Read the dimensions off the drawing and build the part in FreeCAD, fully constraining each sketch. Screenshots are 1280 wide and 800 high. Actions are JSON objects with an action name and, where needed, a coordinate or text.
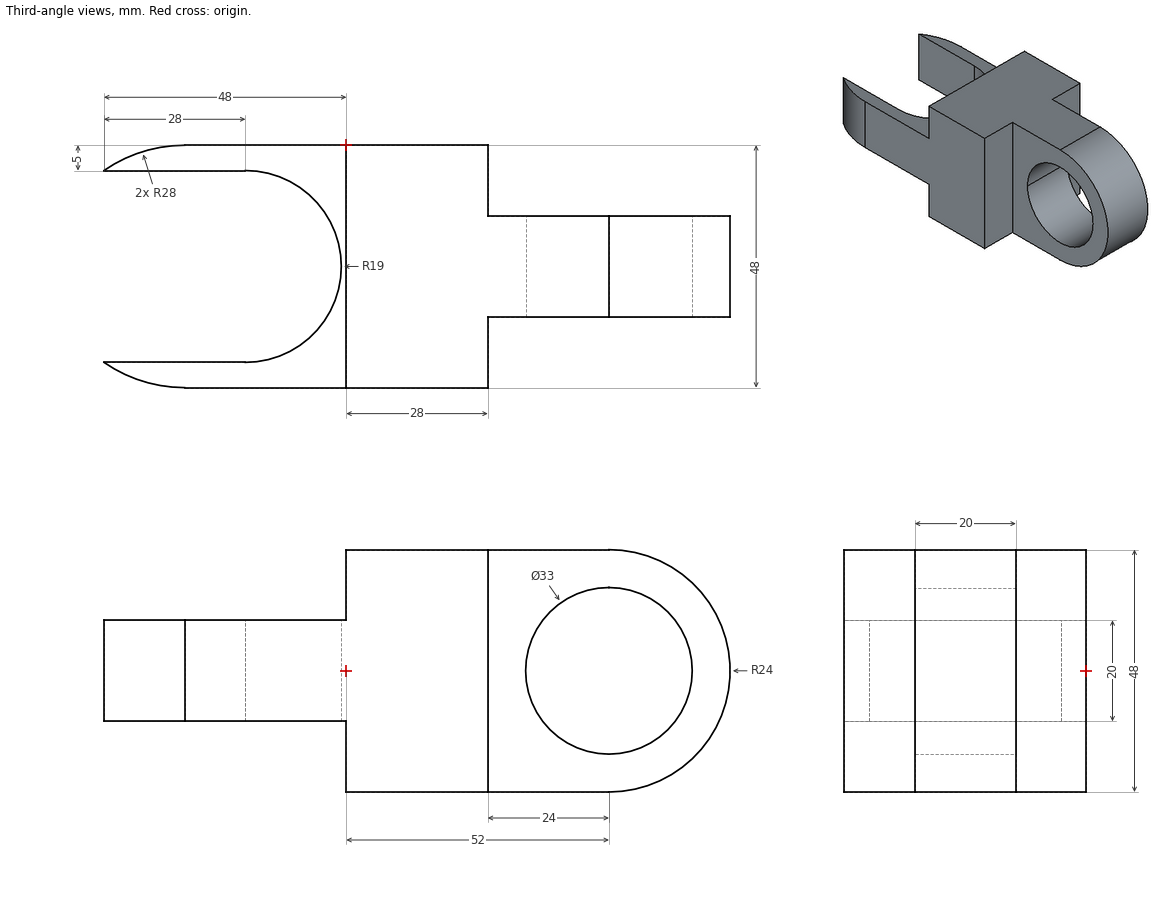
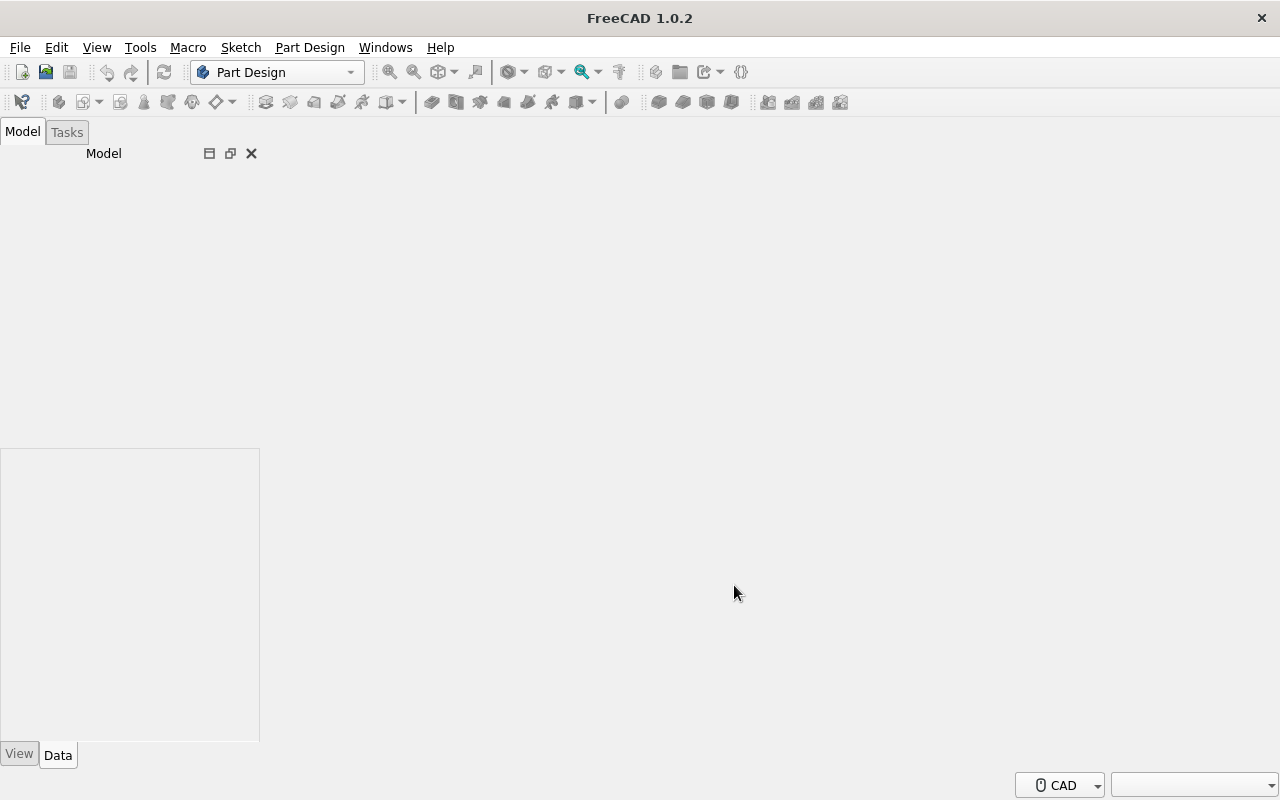
{"action": "left_click", "coordinate": [22, 72]}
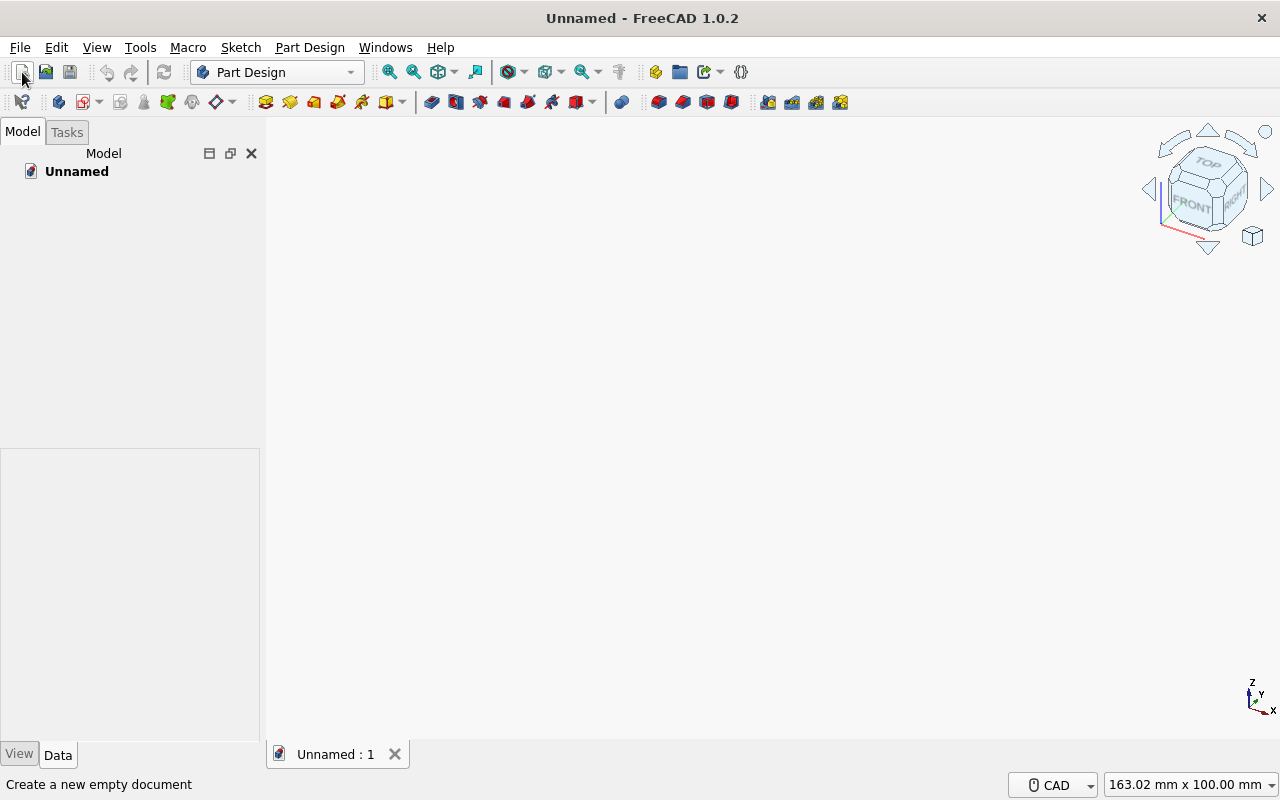
{"action": "left_click", "coordinate": [84, 102]}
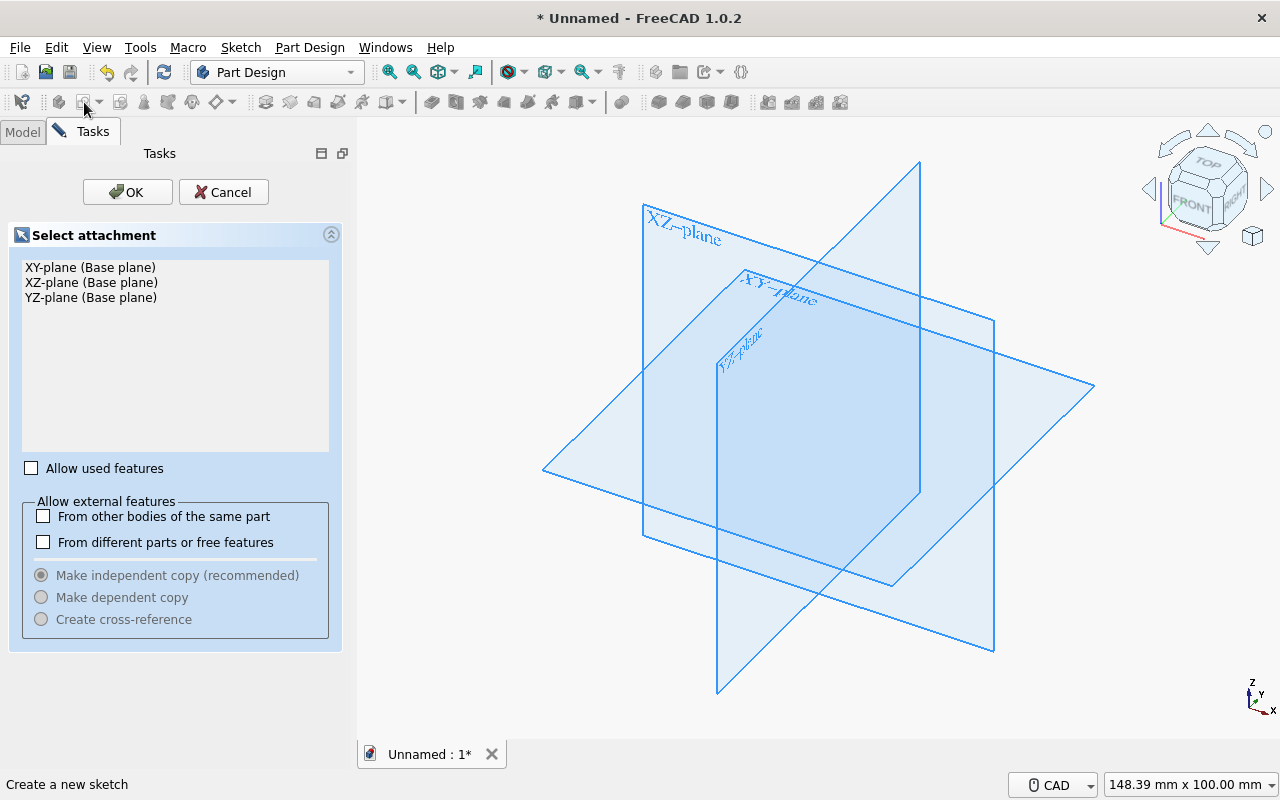
{"action": "left_click", "coordinate": [82, 268]}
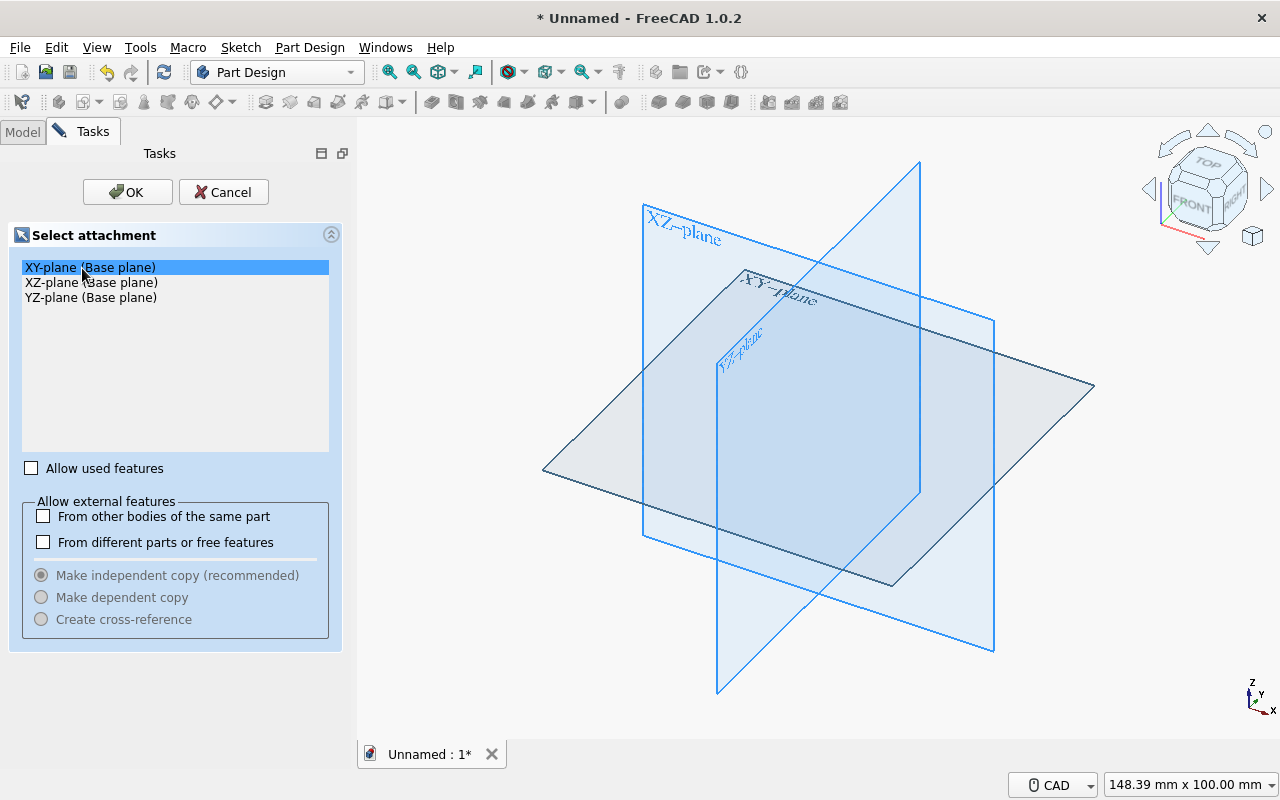
{"action": "left_click", "coordinate": [128, 192]}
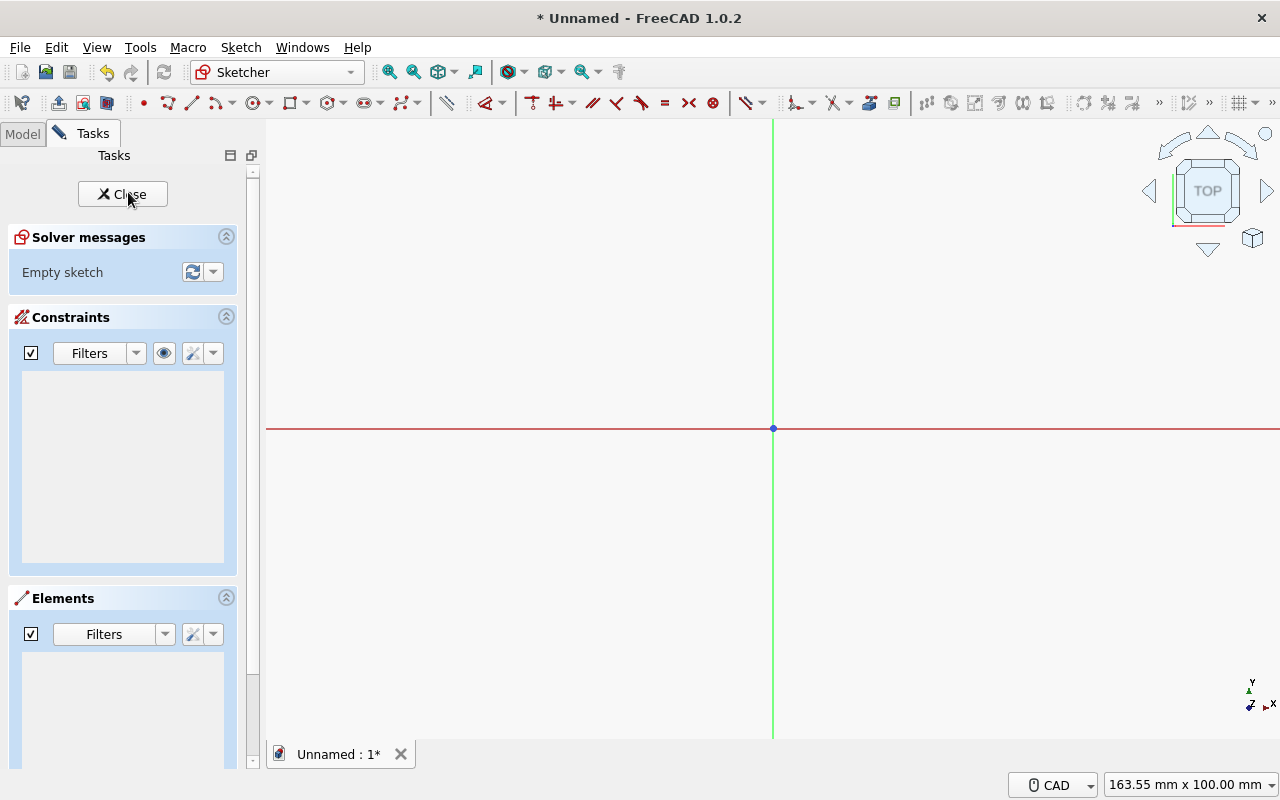
{"action": "scroll", "coordinate": [294, 147], "scroll_direction": "down", "scroll_amount": 1}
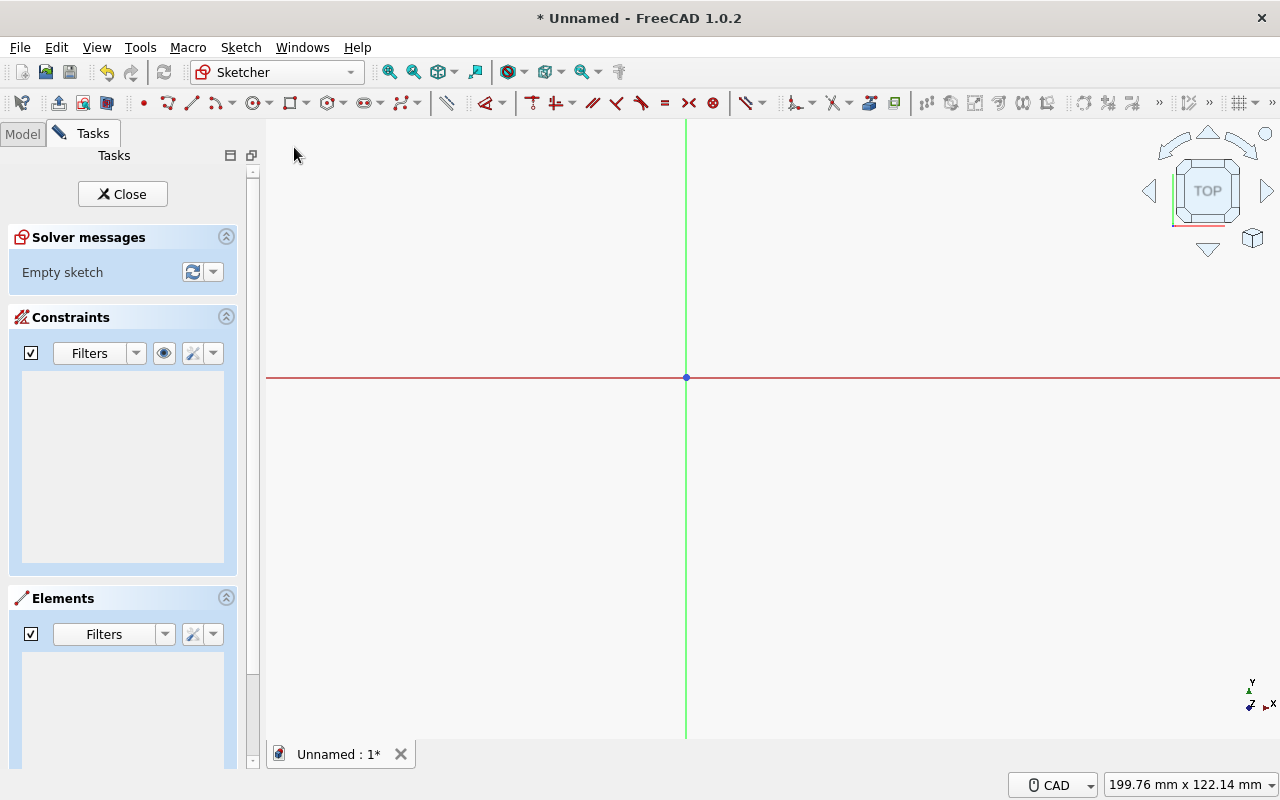
{"action": "scroll", "coordinate": [864, 644], "scroll_direction": "up", "scroll_amount": 2}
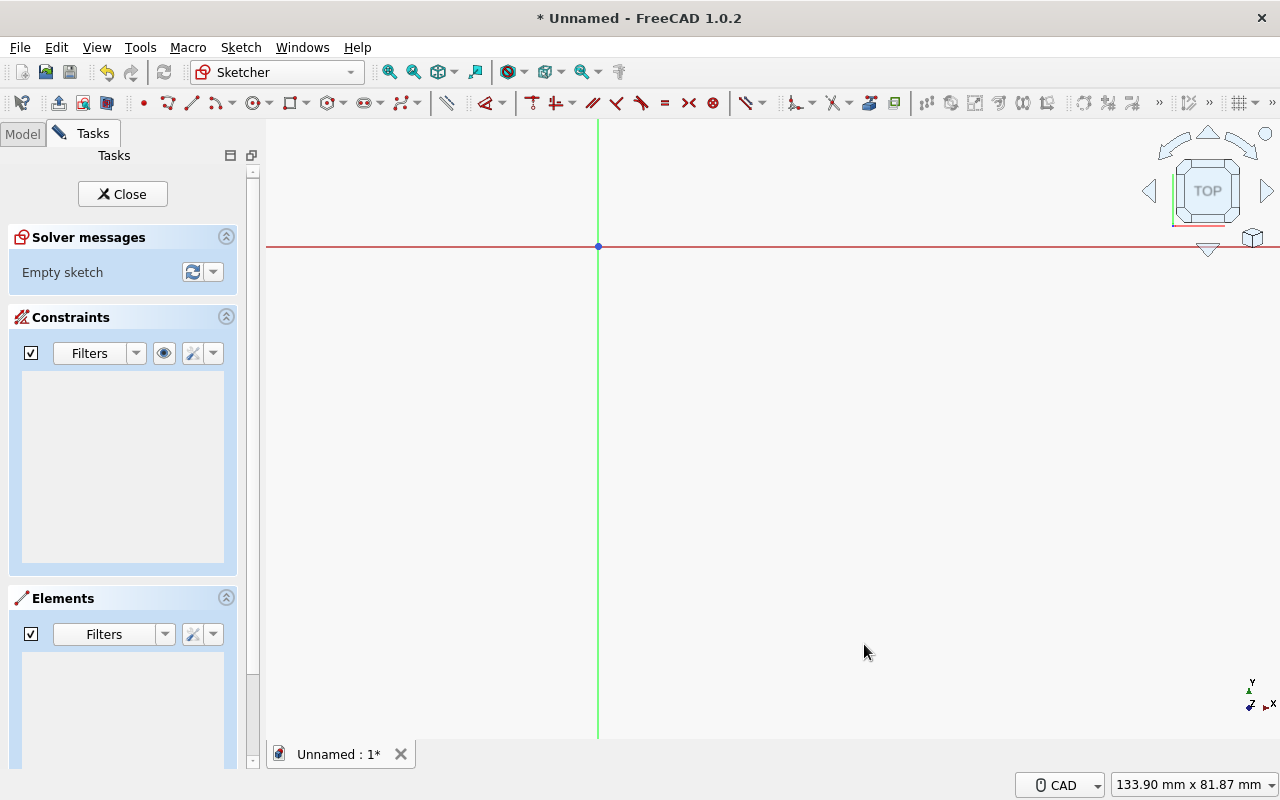
{"action": "left_click", "coordinate": [290, 104]}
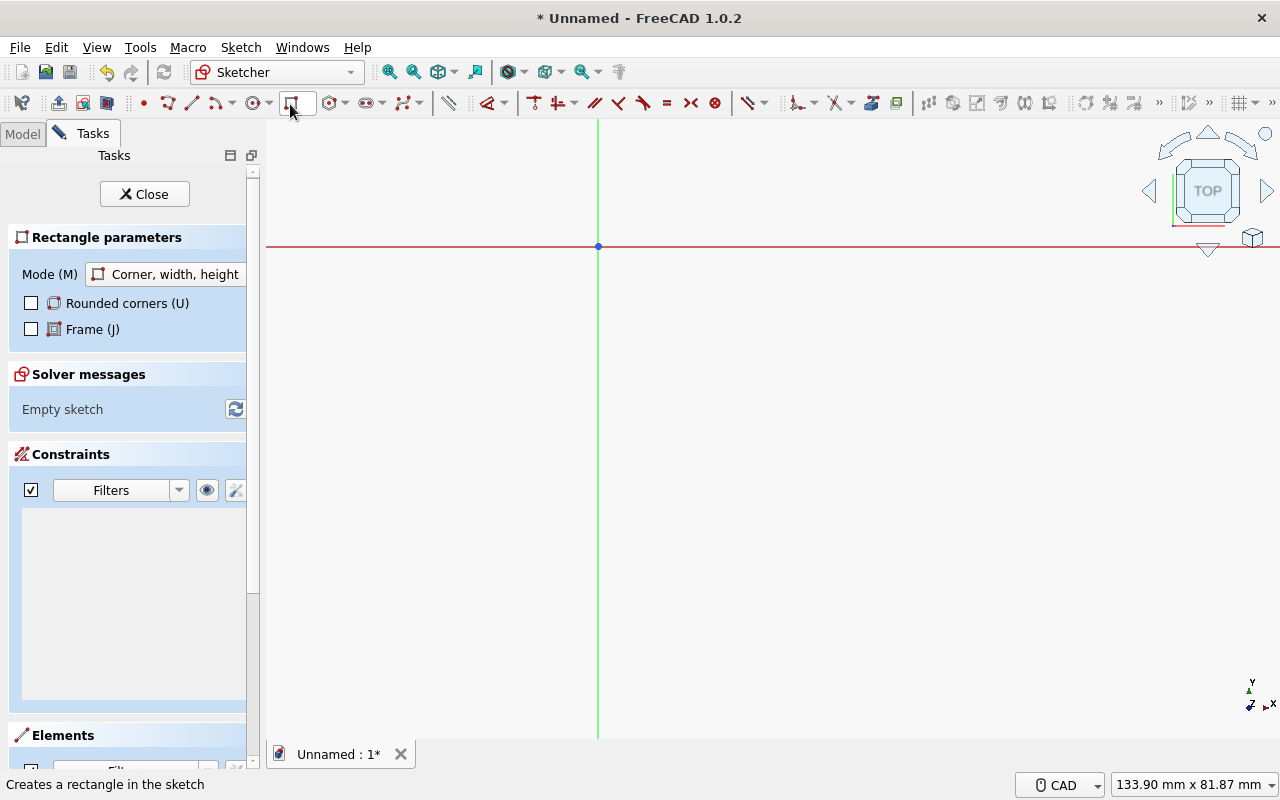
{"action": "left_click", "coordinate": [598, 247]}
{"action": "mouse_move", "coordinate": [810, 610]}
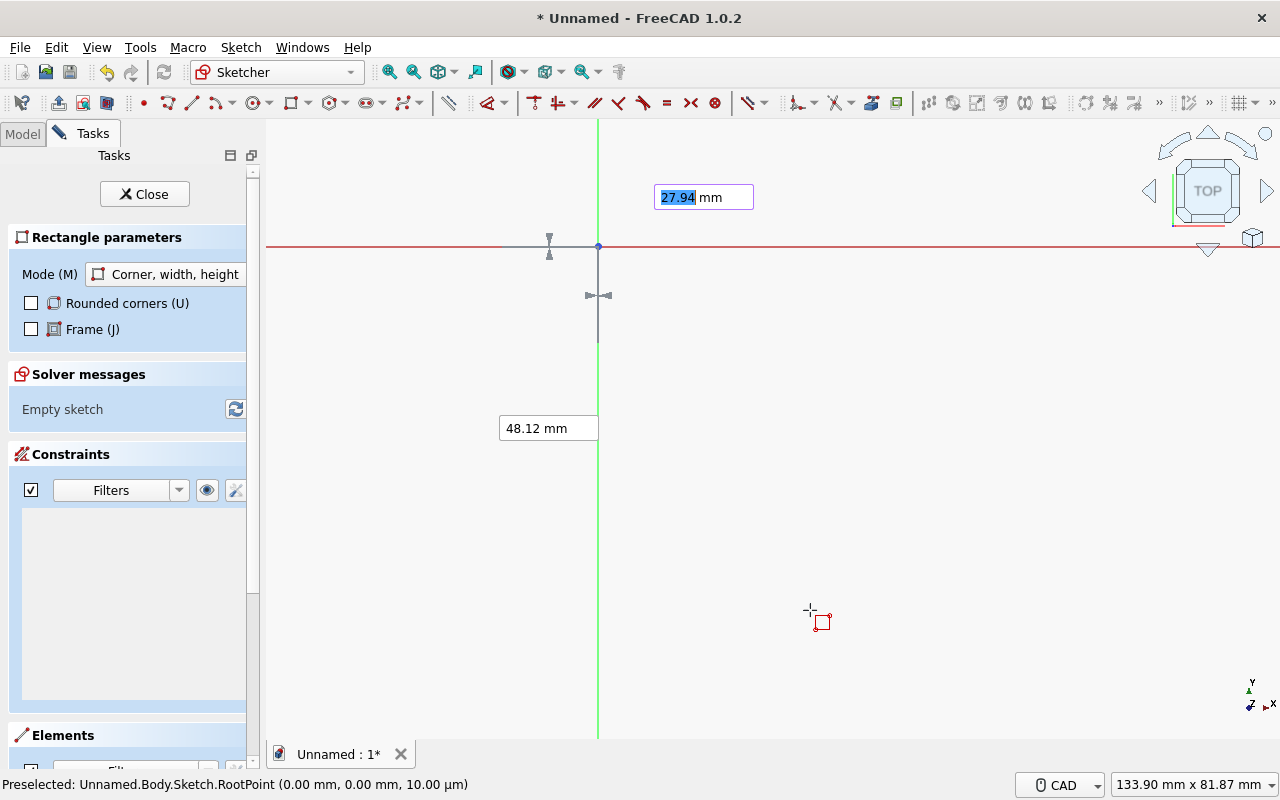
{"action": "type", "text": "28"}
{"action": "key", "text": "Tab"}
{"action": "type", "text": "48"}
{"action": "key", "text": "Return"}
{"action": "key", "text": "Escape"}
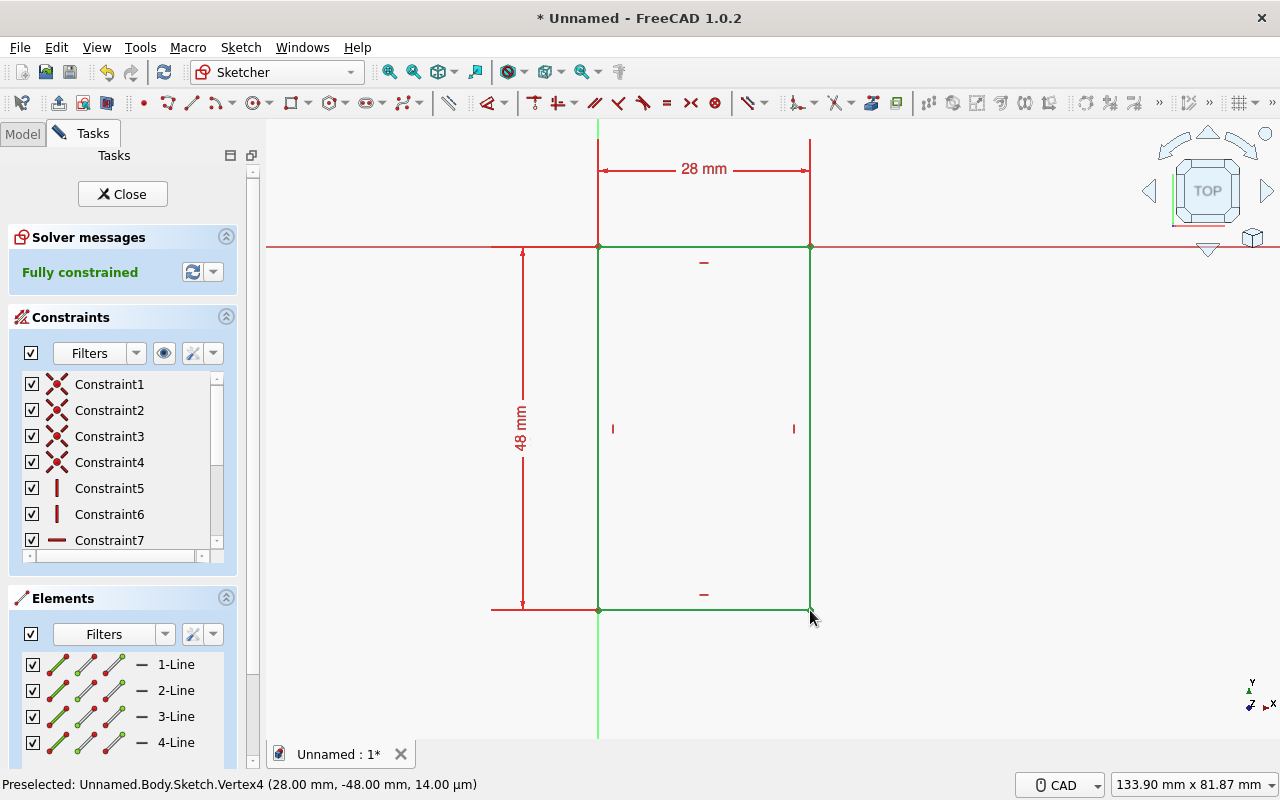
{"action": "left_click", "coordinate": [123, 194]}